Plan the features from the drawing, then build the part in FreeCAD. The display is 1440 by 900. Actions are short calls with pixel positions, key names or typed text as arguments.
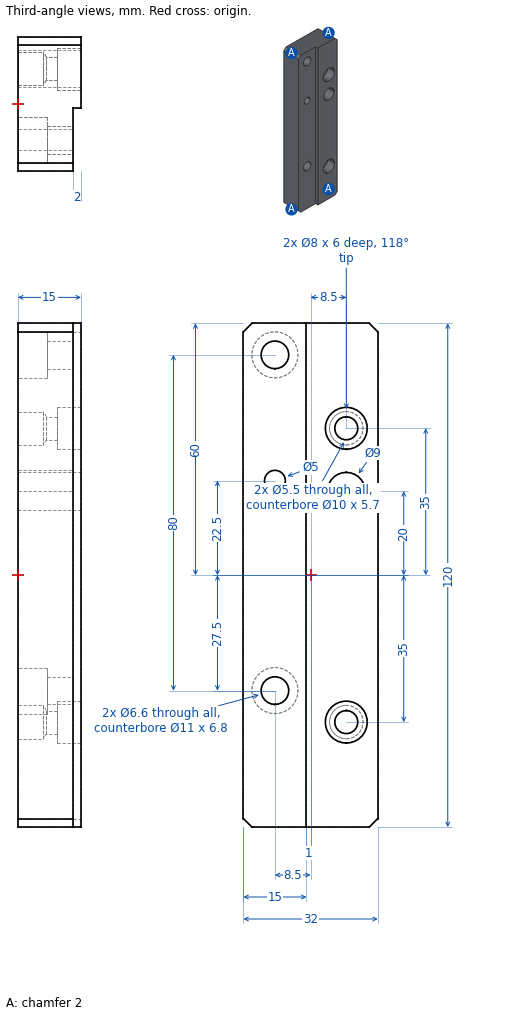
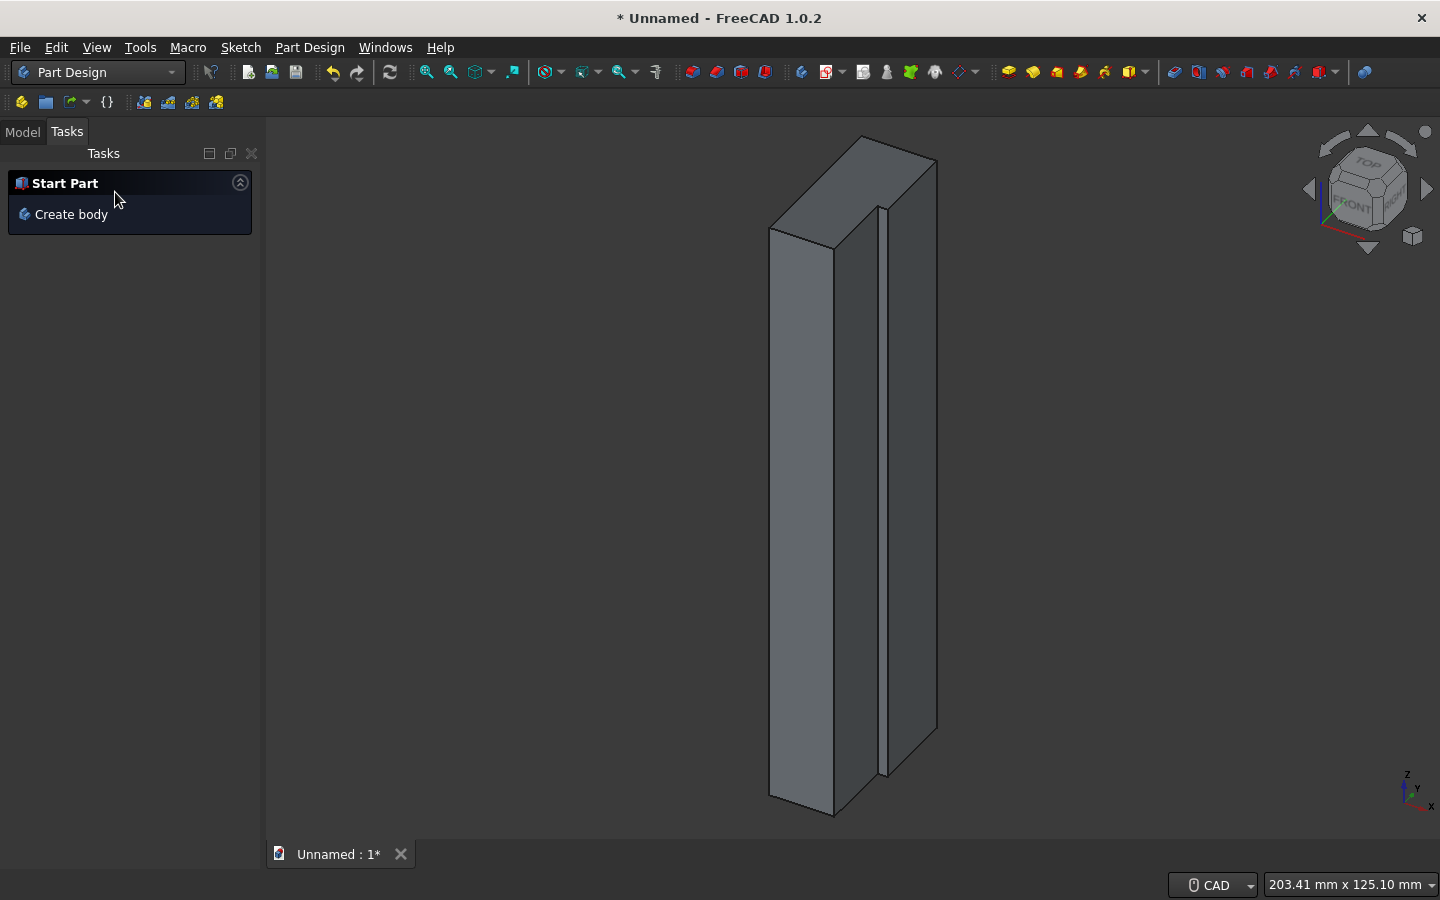
click(826, 72)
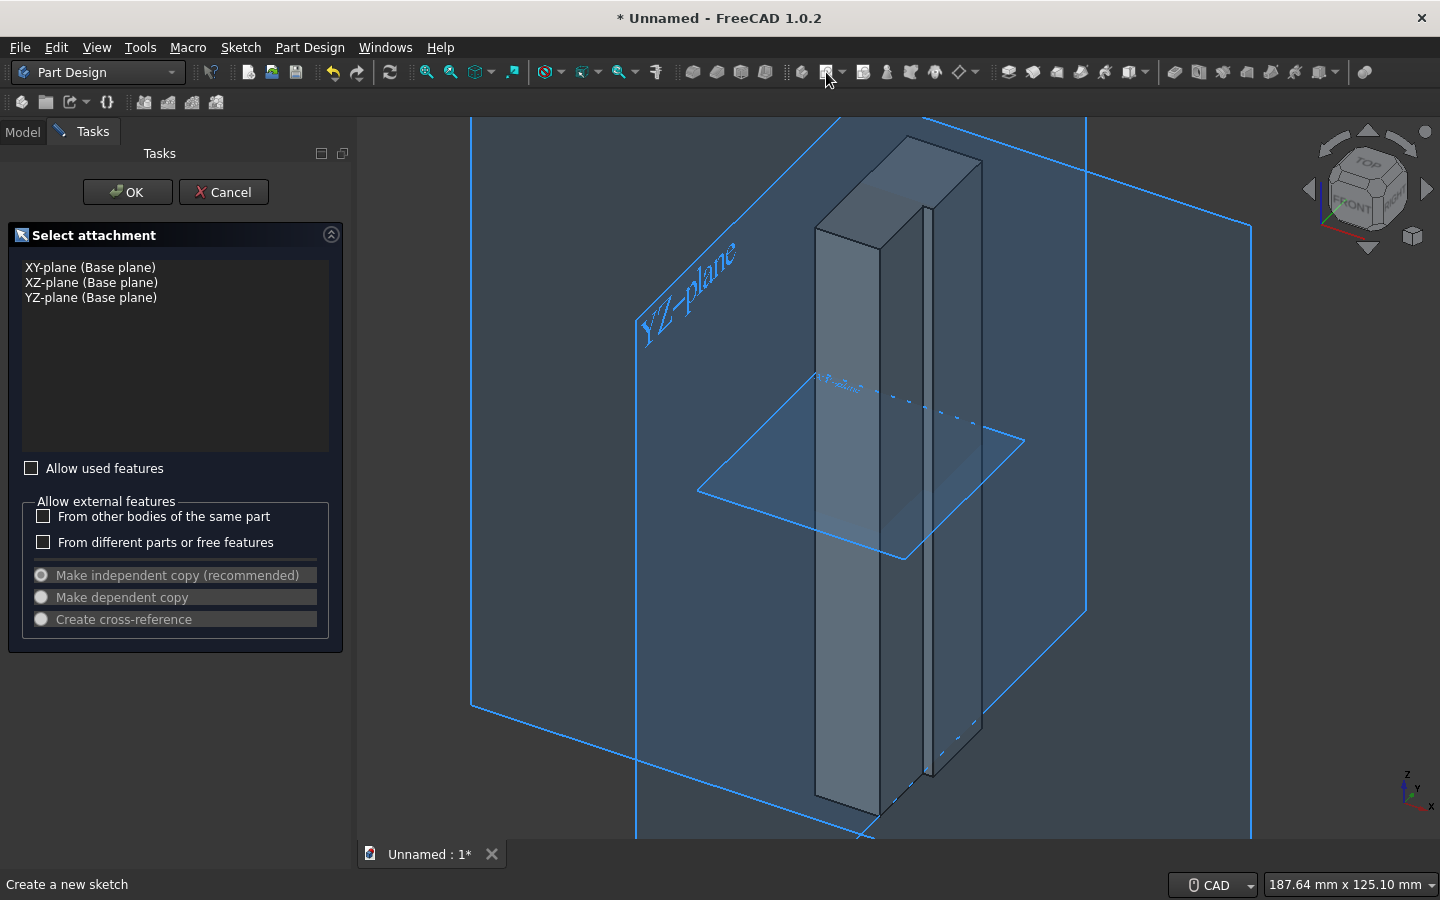
click(82, 298)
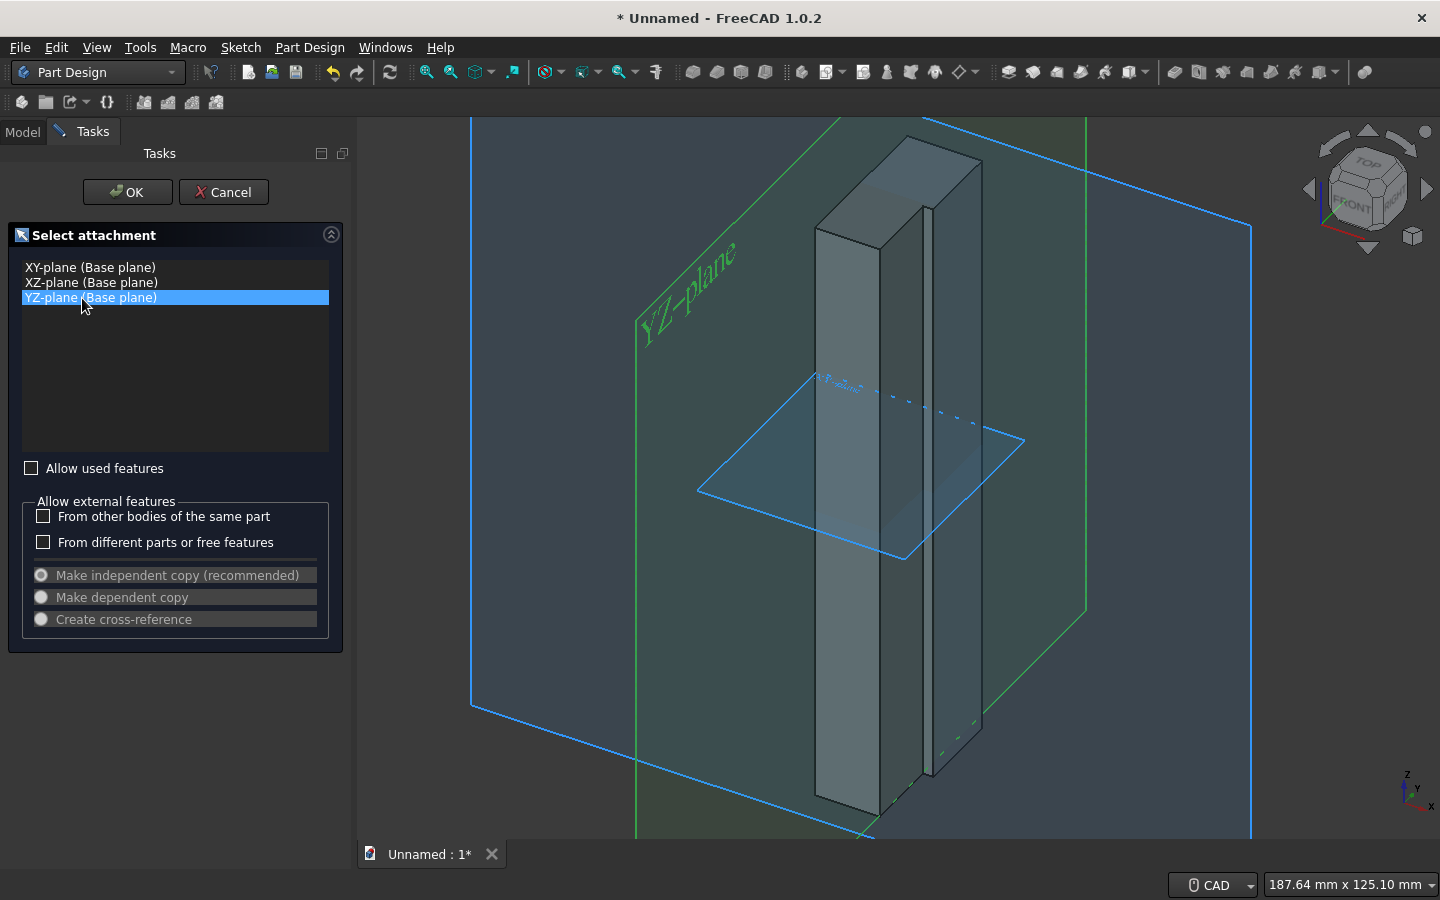
click(128, 192)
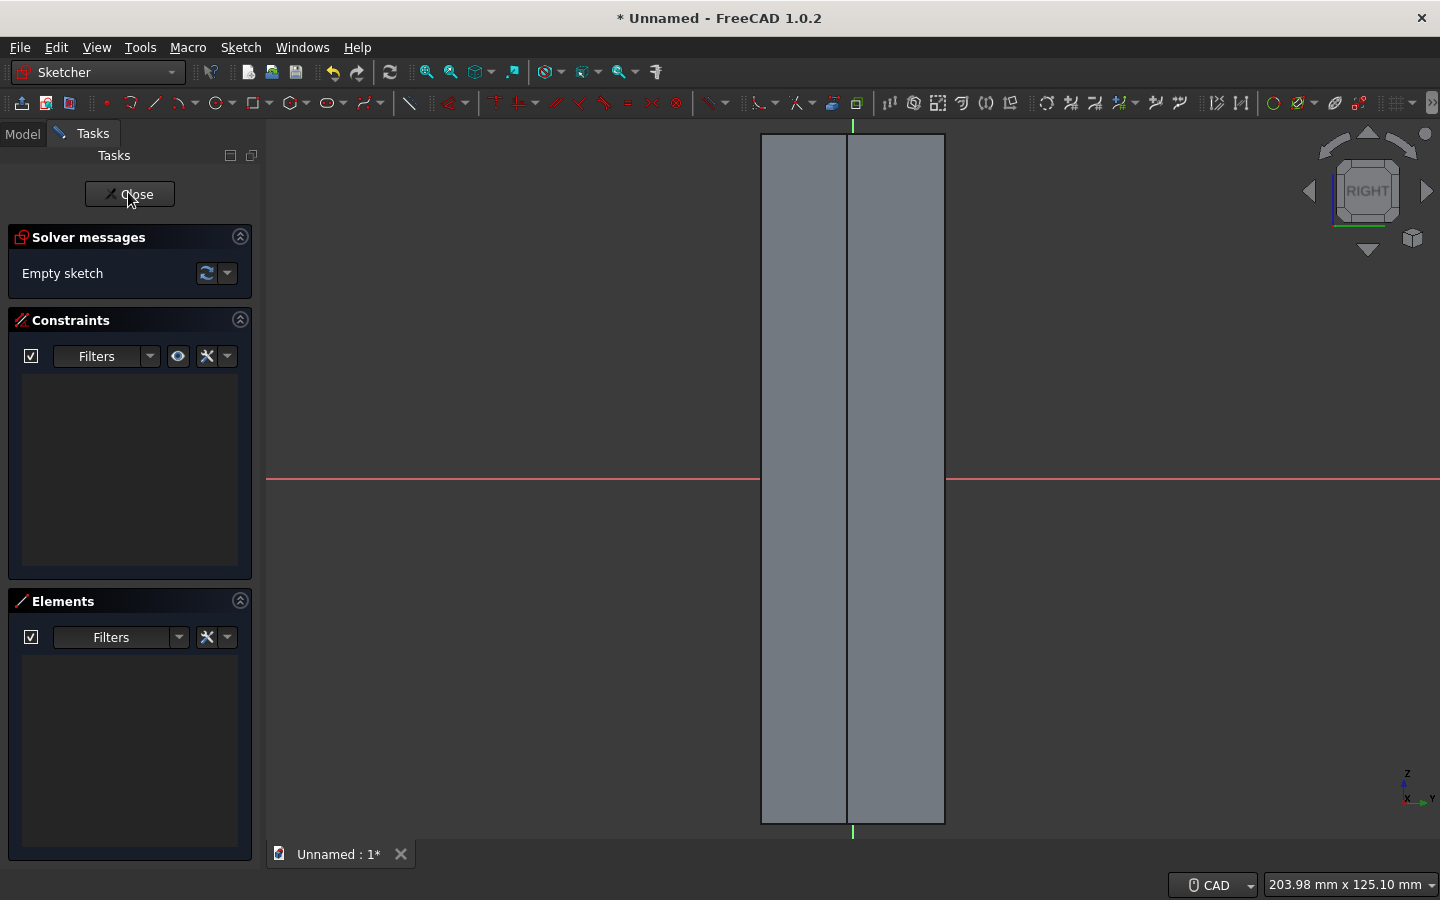
click(70, 104)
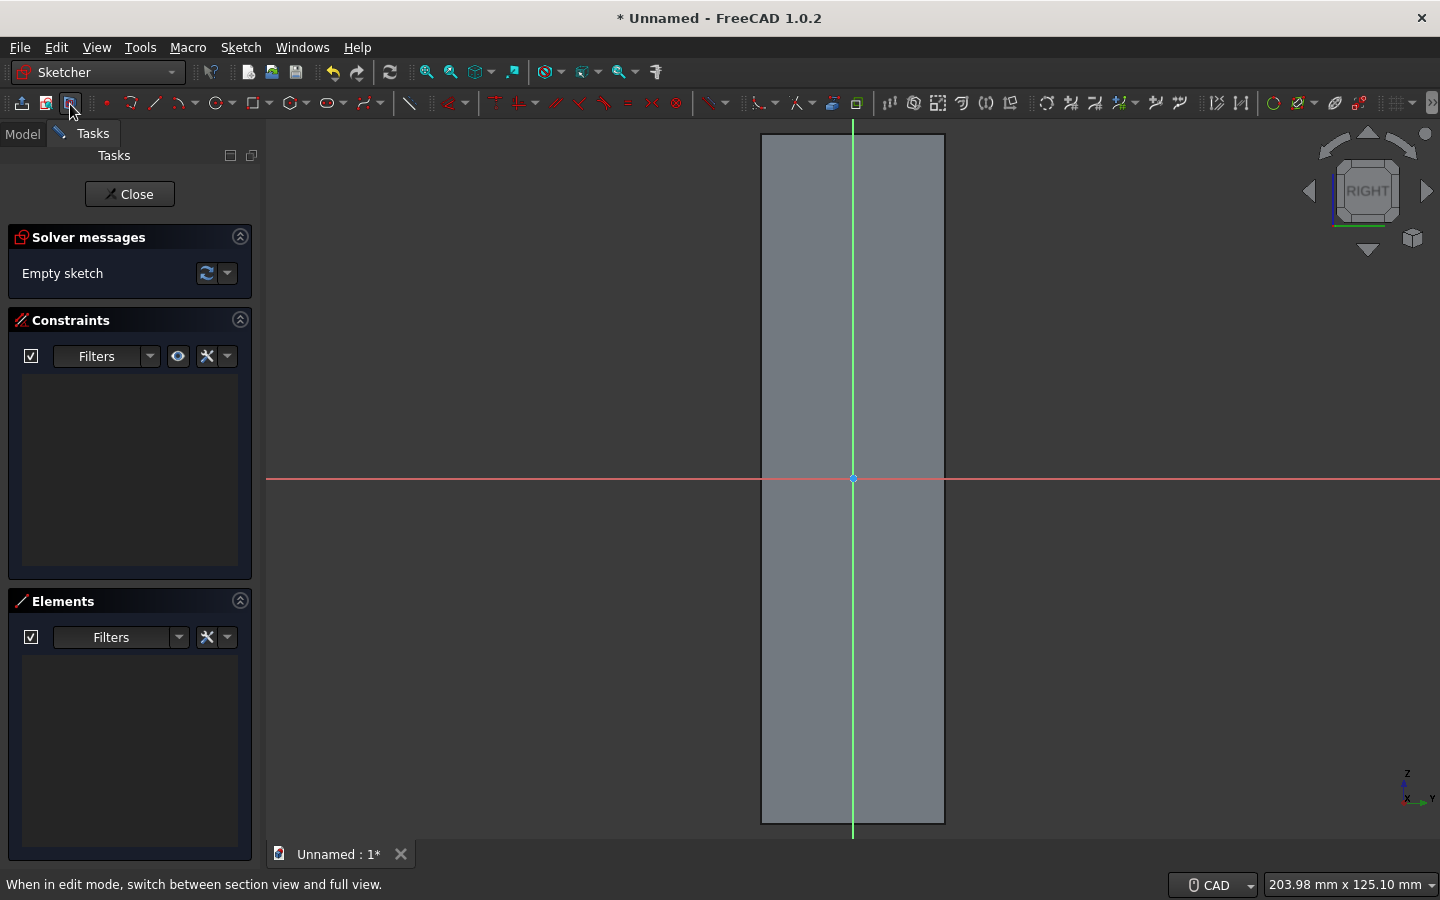
click(216, 104)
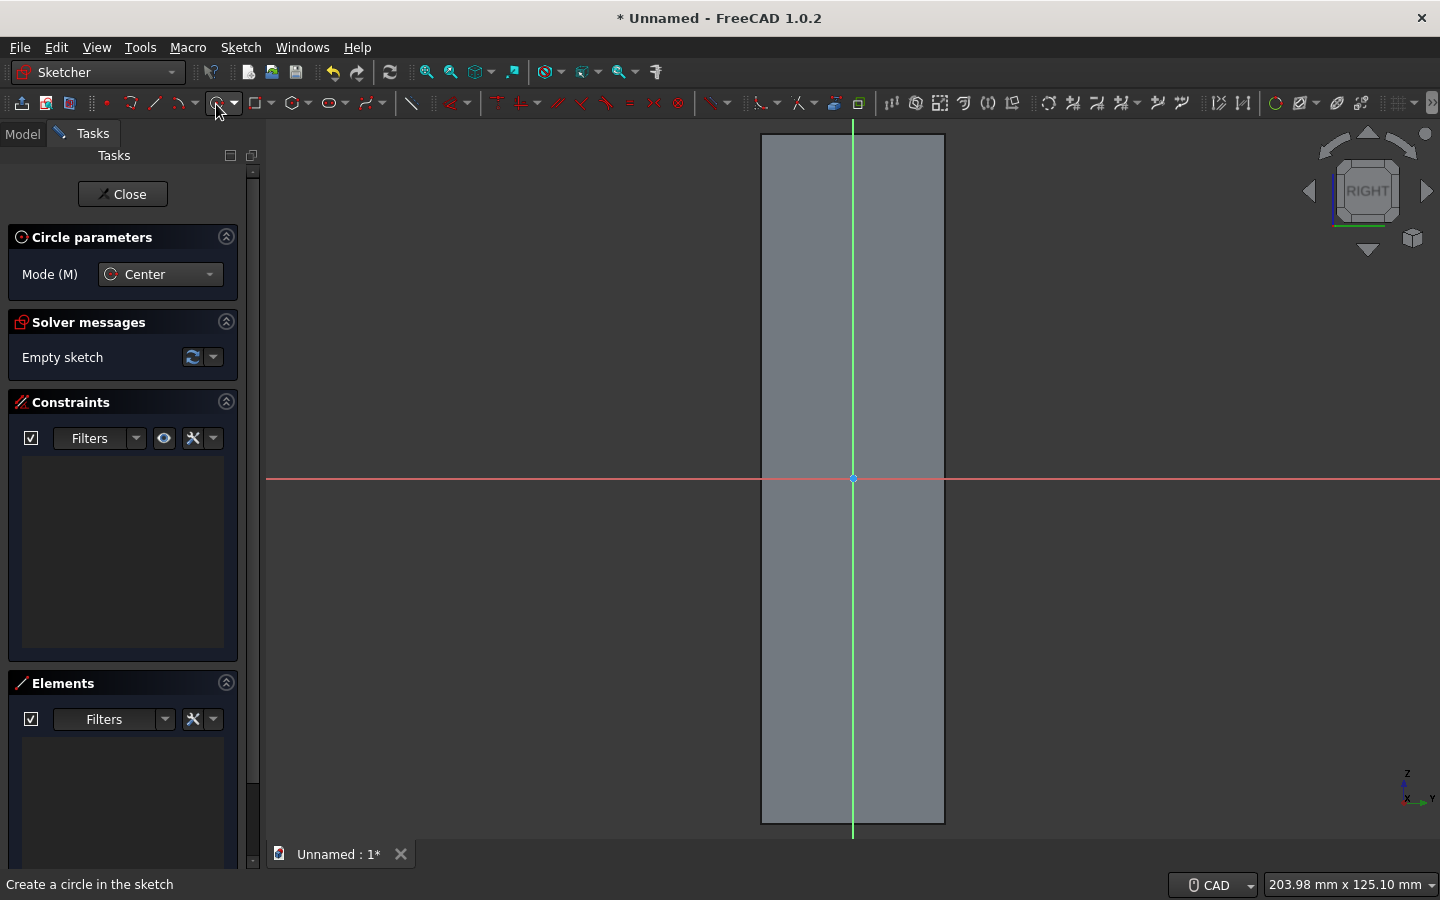
click(902, 278)
click(918, 261)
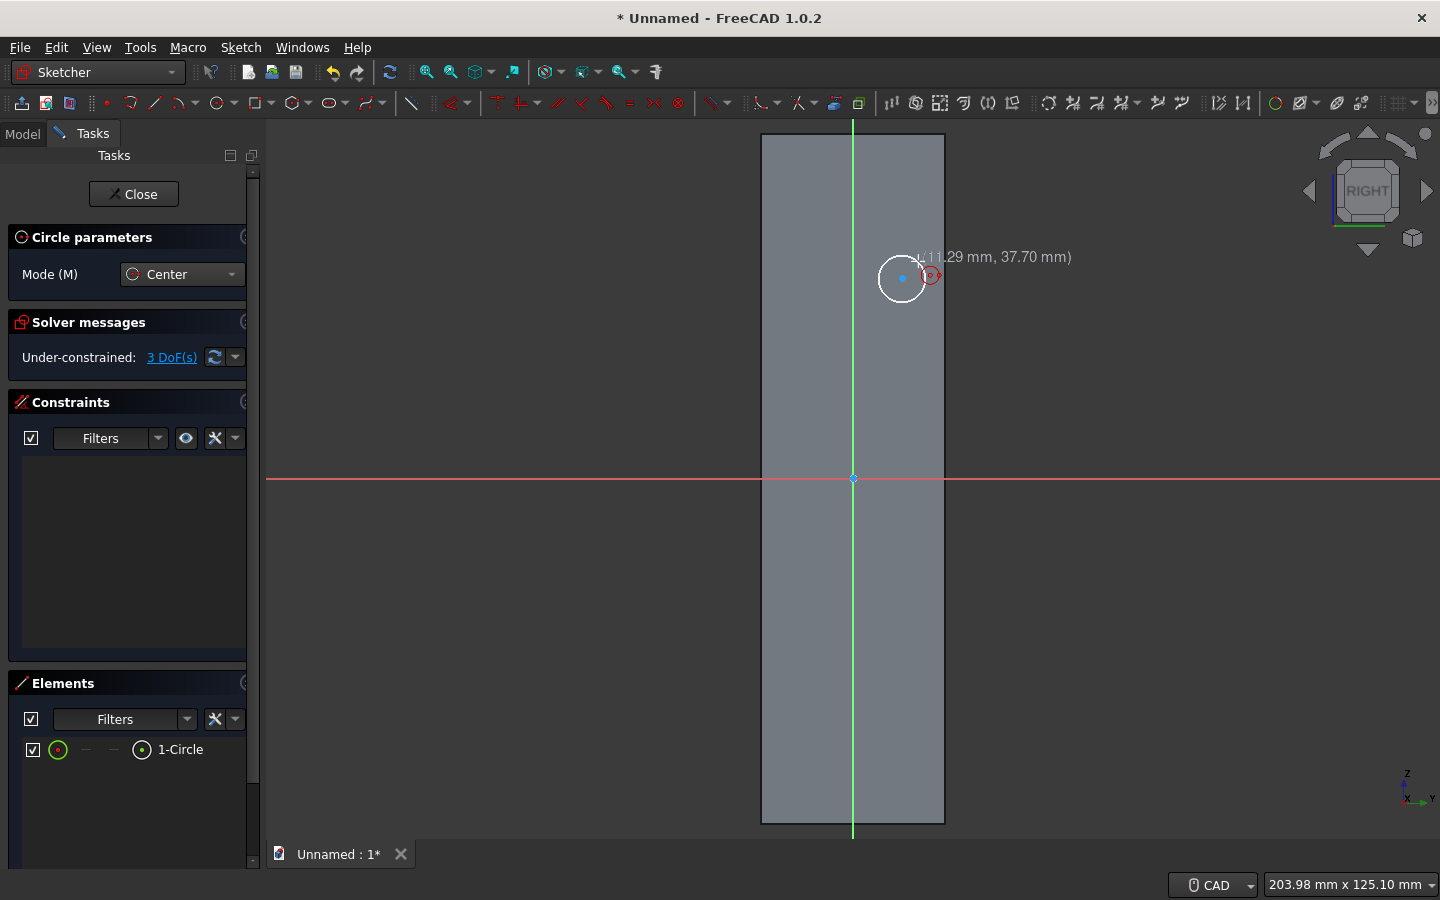
click(902, 680)
click(918, 664)
key(Escape)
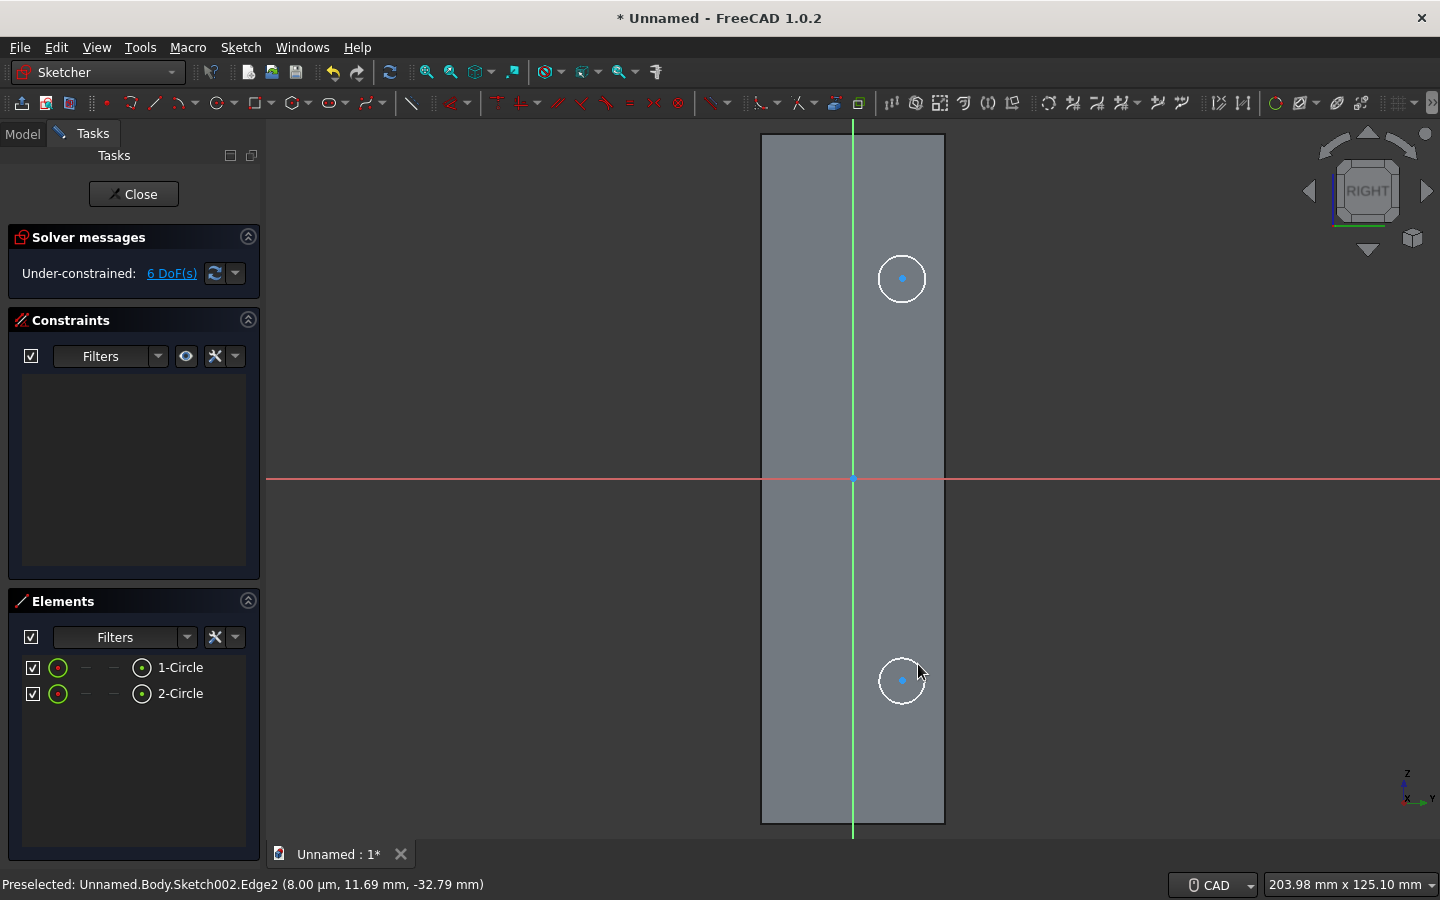
click(918, 262)